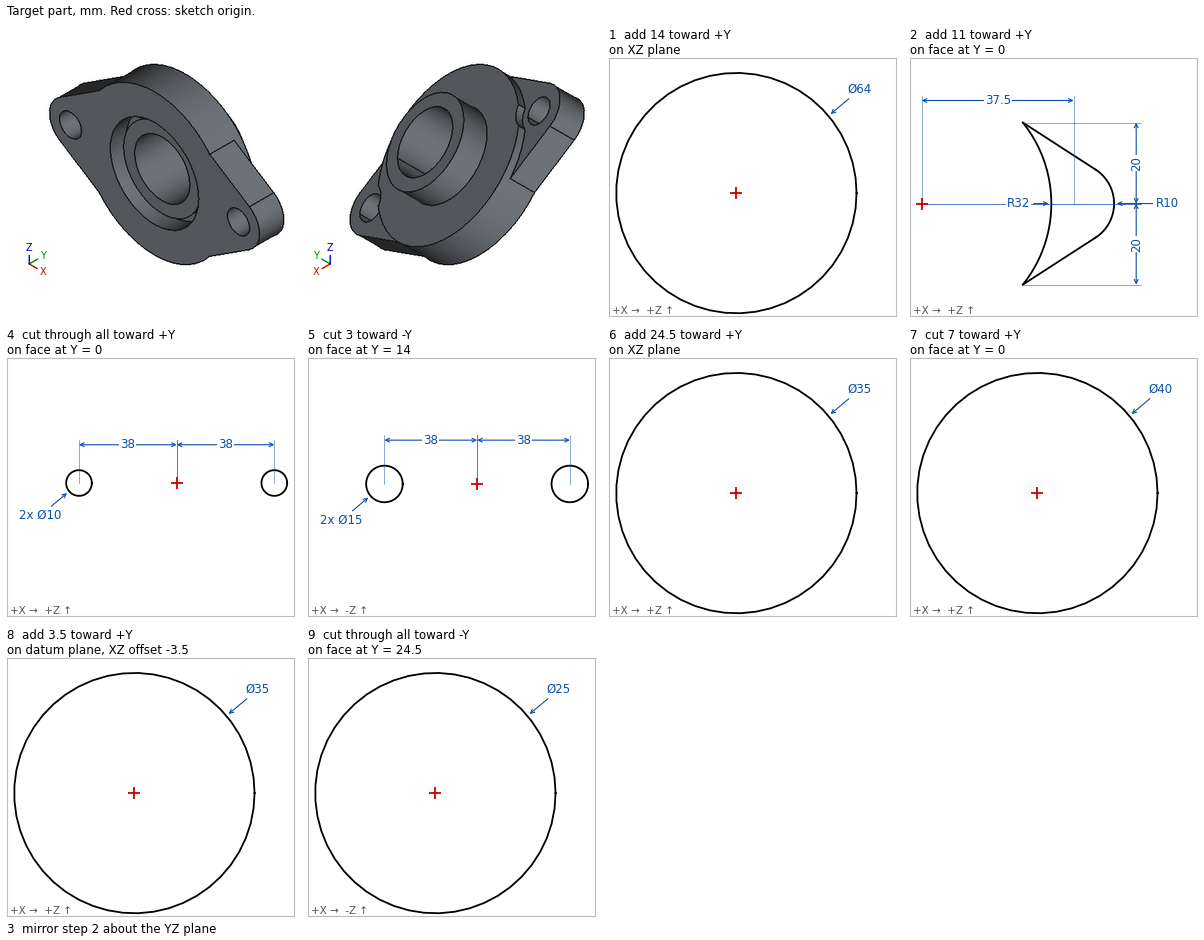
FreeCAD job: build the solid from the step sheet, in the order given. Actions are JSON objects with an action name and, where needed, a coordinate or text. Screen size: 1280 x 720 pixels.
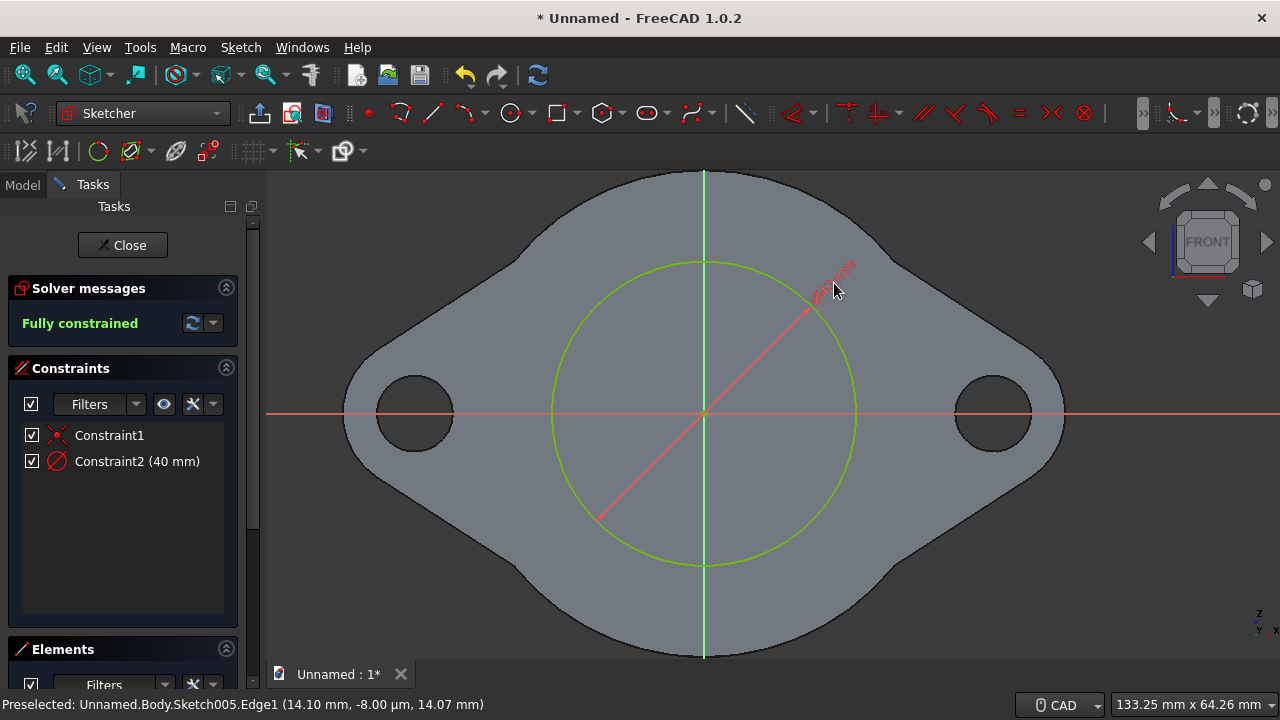
{"action": "left_click", "coordinate": [123, 245]}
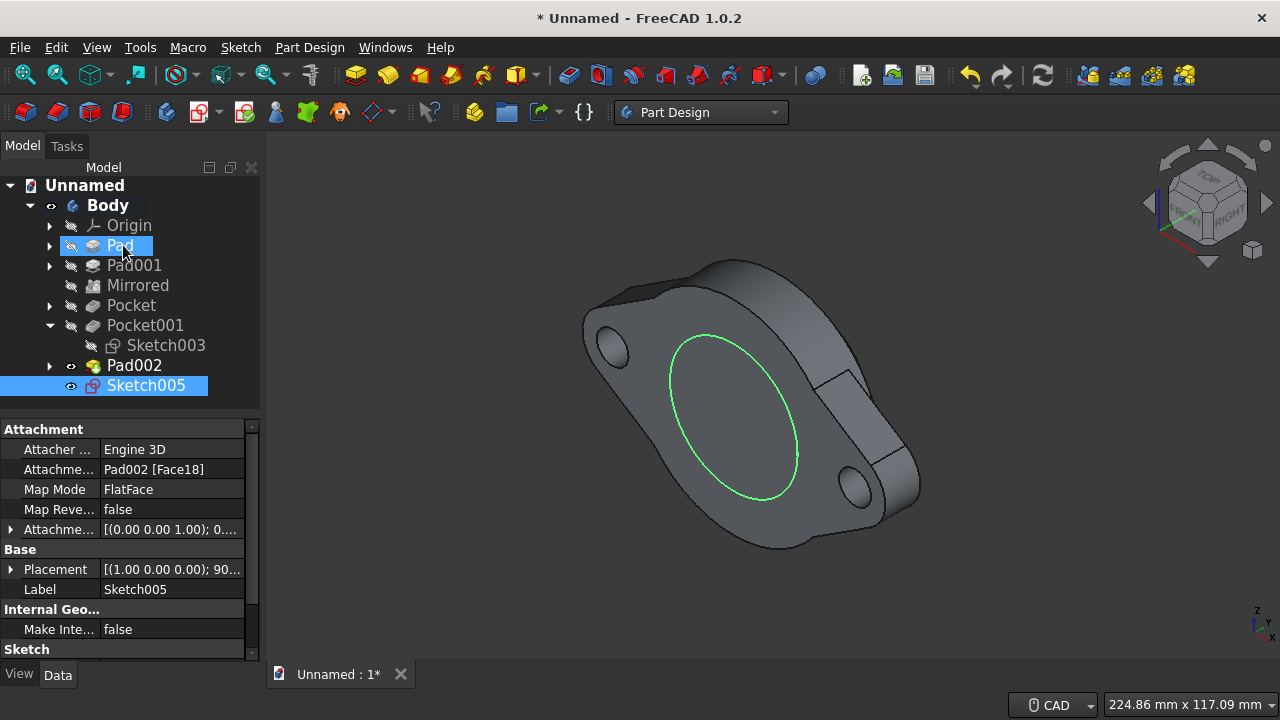
{"action": "left_click", "coordinate": [570, 76]}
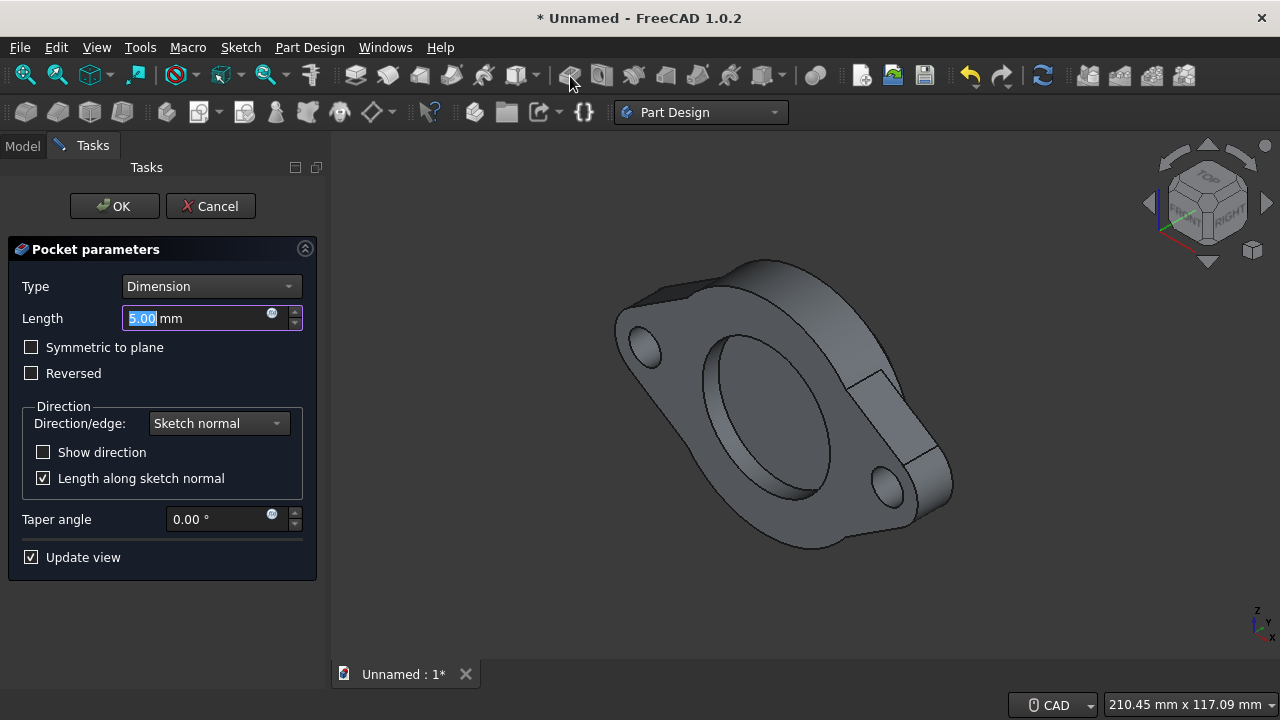
{"action": "type", "text": "7"}
{"action": "key", "text": "Tab"}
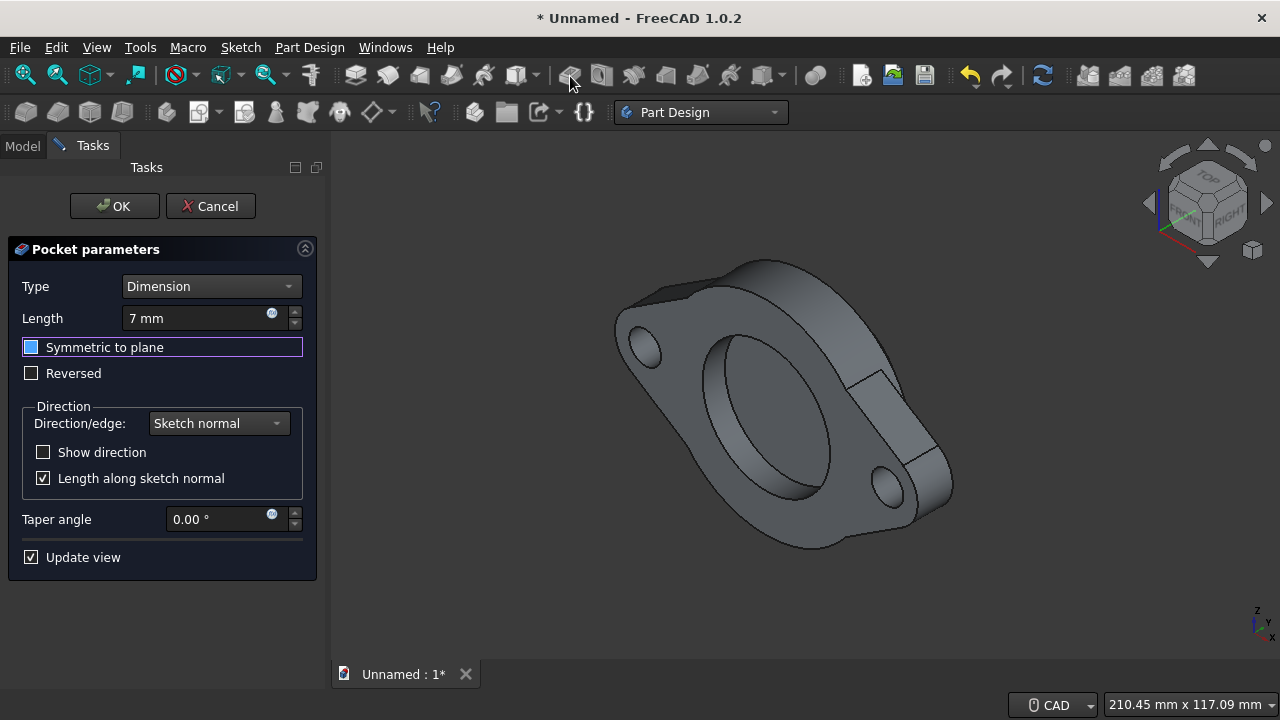
{"action": "left_click", "coordinate": [115, 206]}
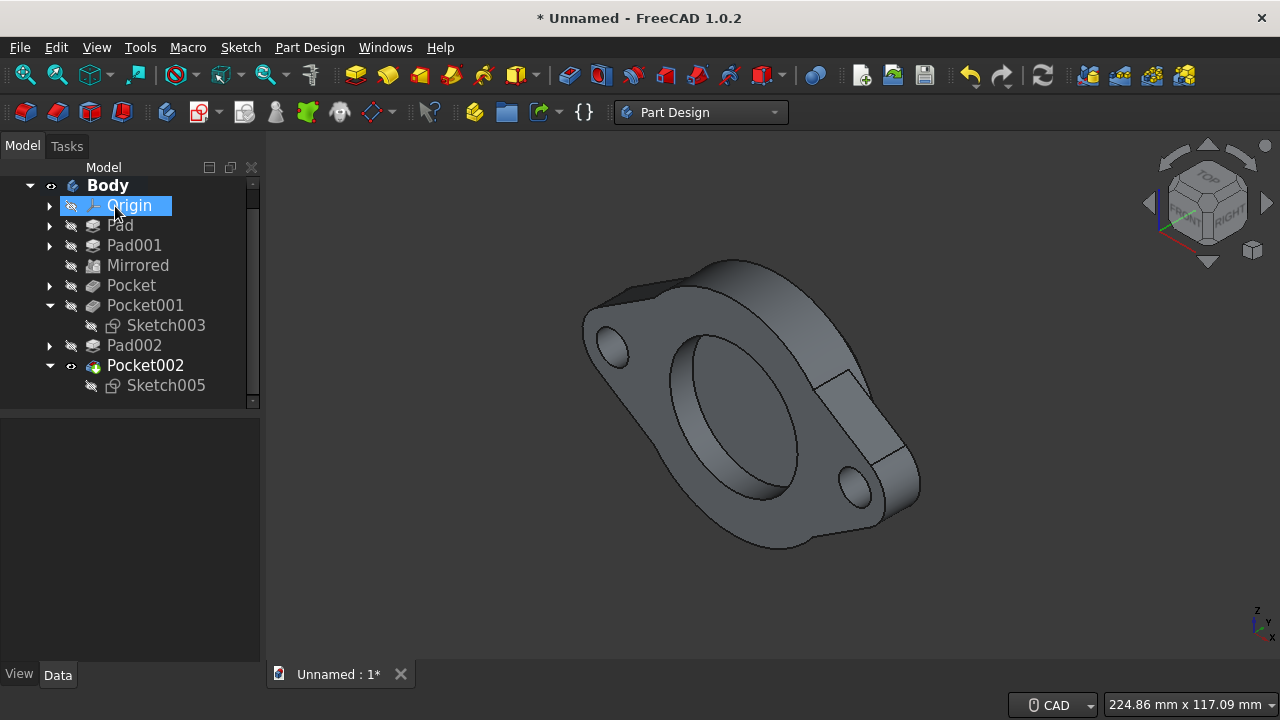
{"action": "left_click", "coordinate": [50, 206]}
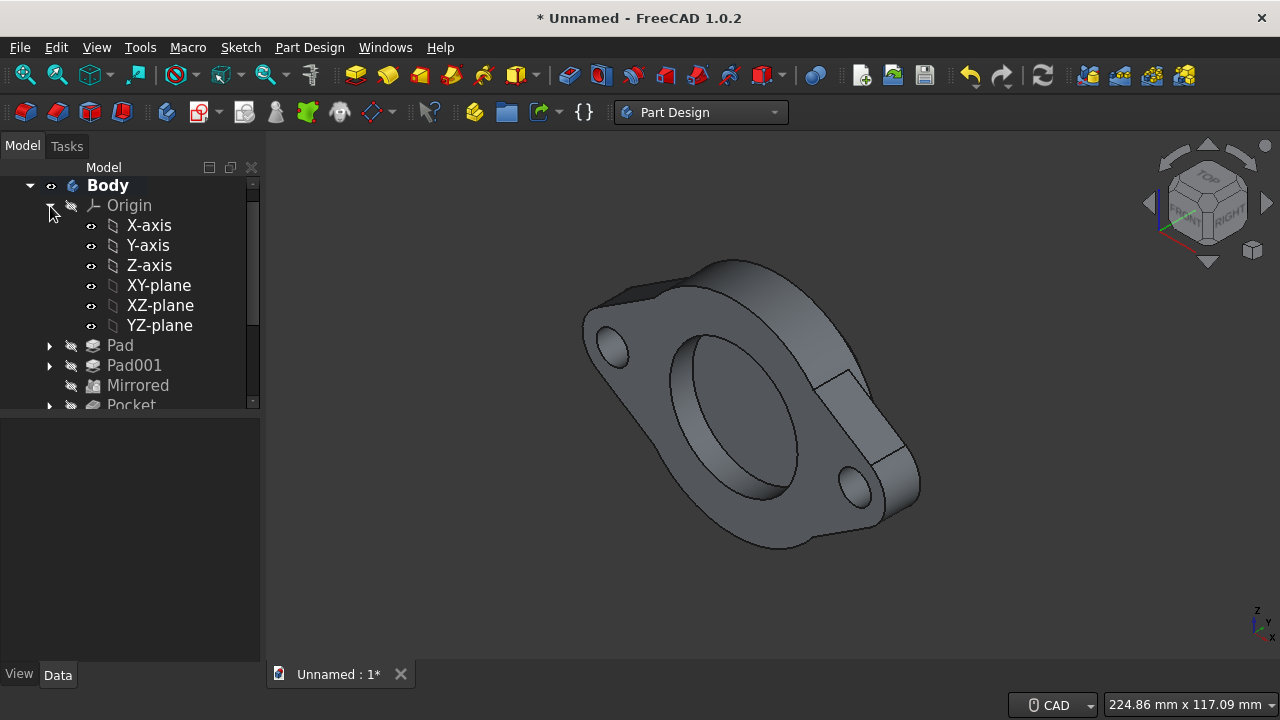
{"action": "left_click", "coordinate": [136, 306]}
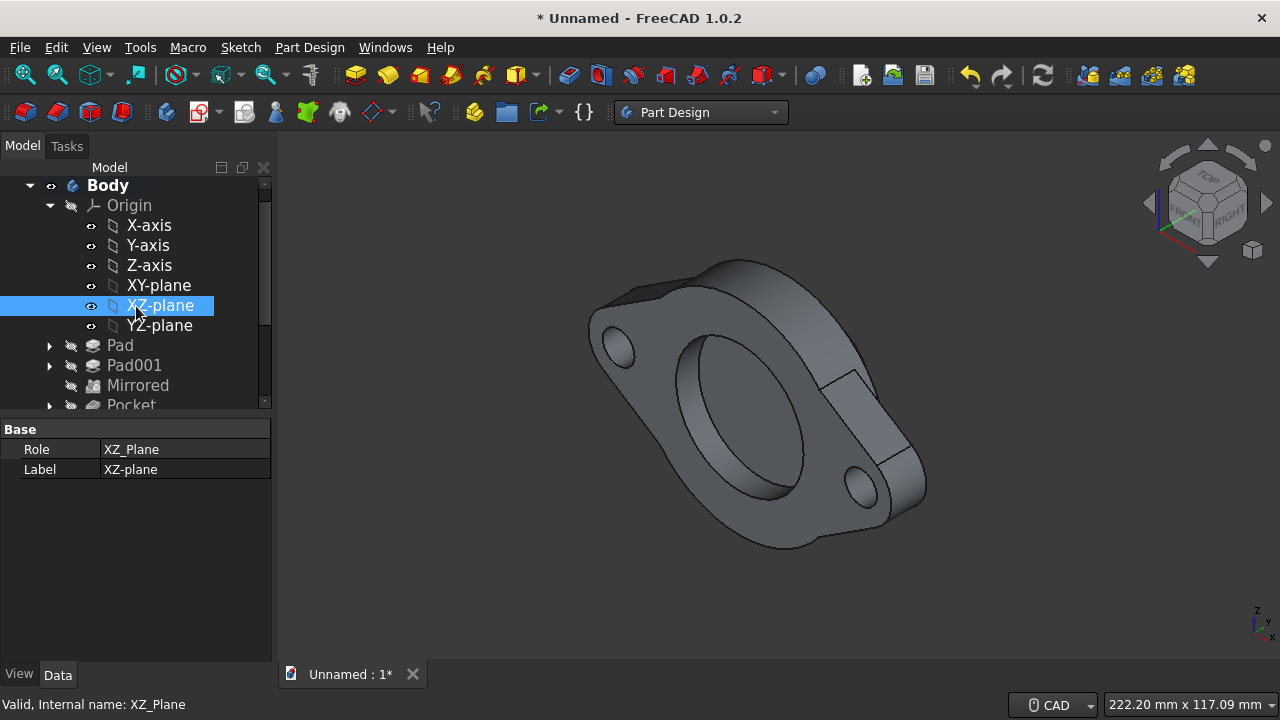
{"action": "left_click", "coordinate": [372, 112]}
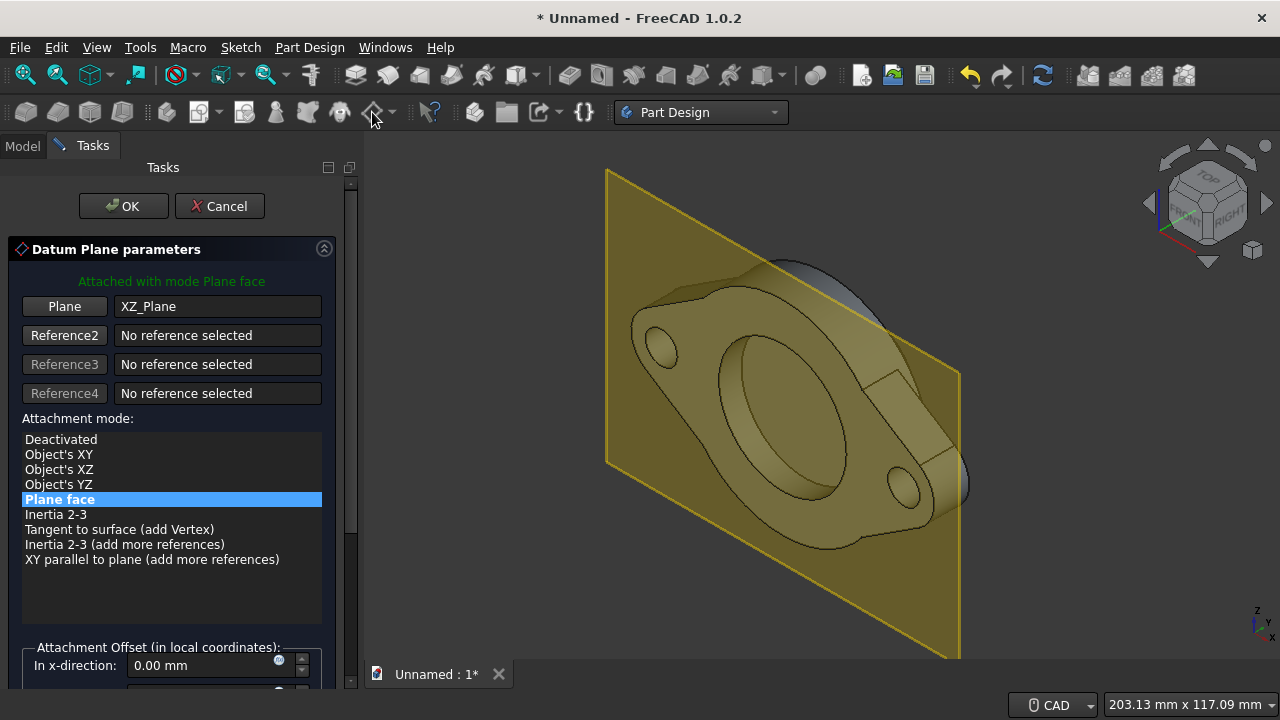
{"action": "scroll", "coordinate": [351, 432], "scroll_direction": "down", "scroll_amount": 2}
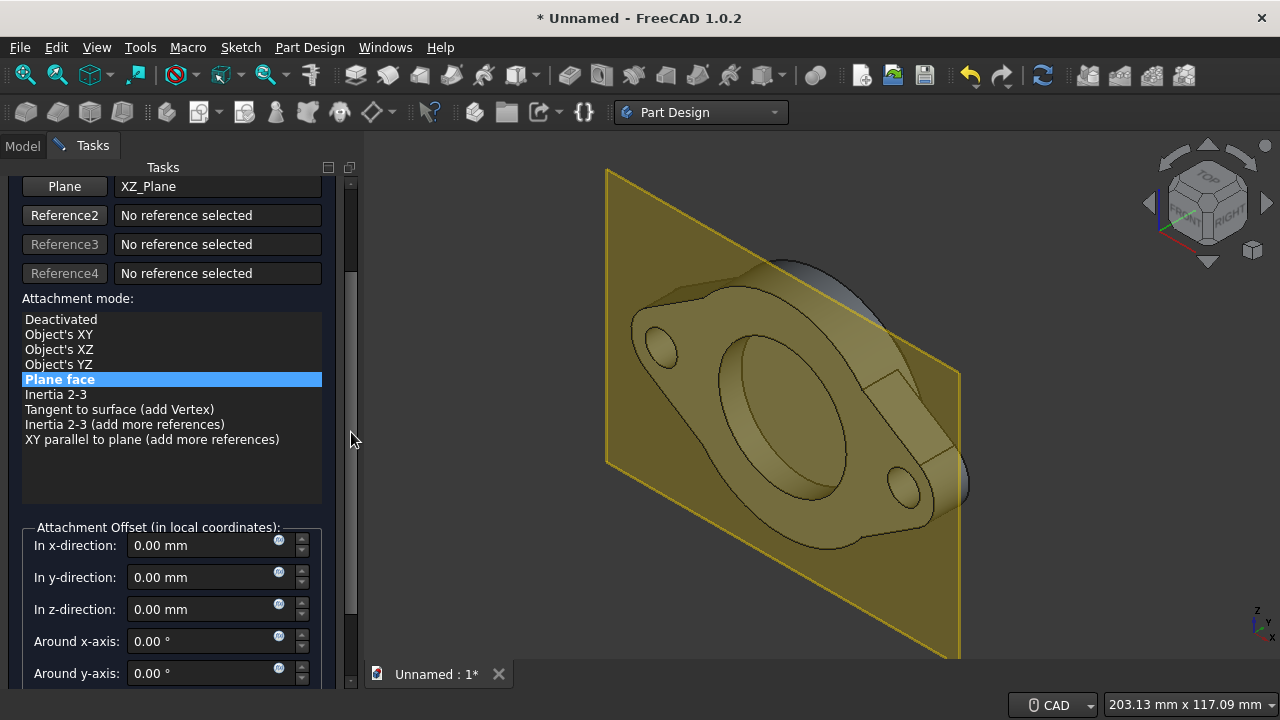
{"action": "triple_click", "coordinate": [210, 609]}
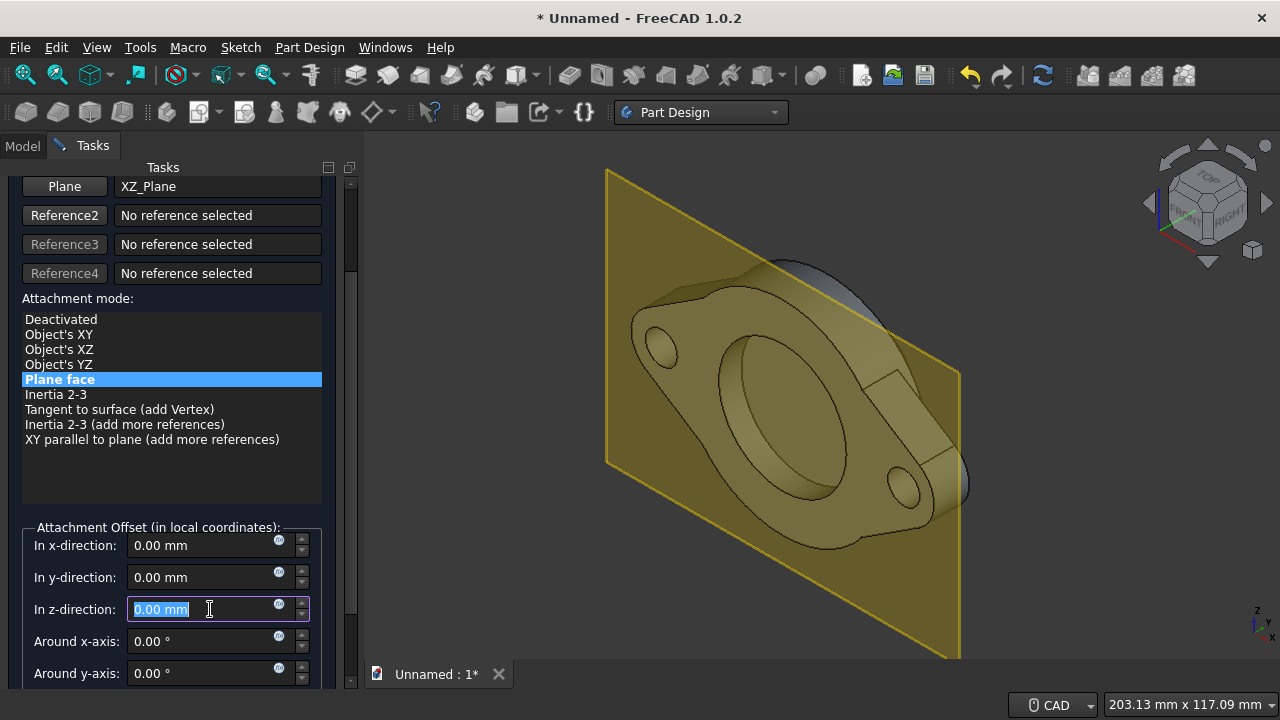
{"action": "type", "text": "-3.5"}
{"action": "key", "text": "Tab"}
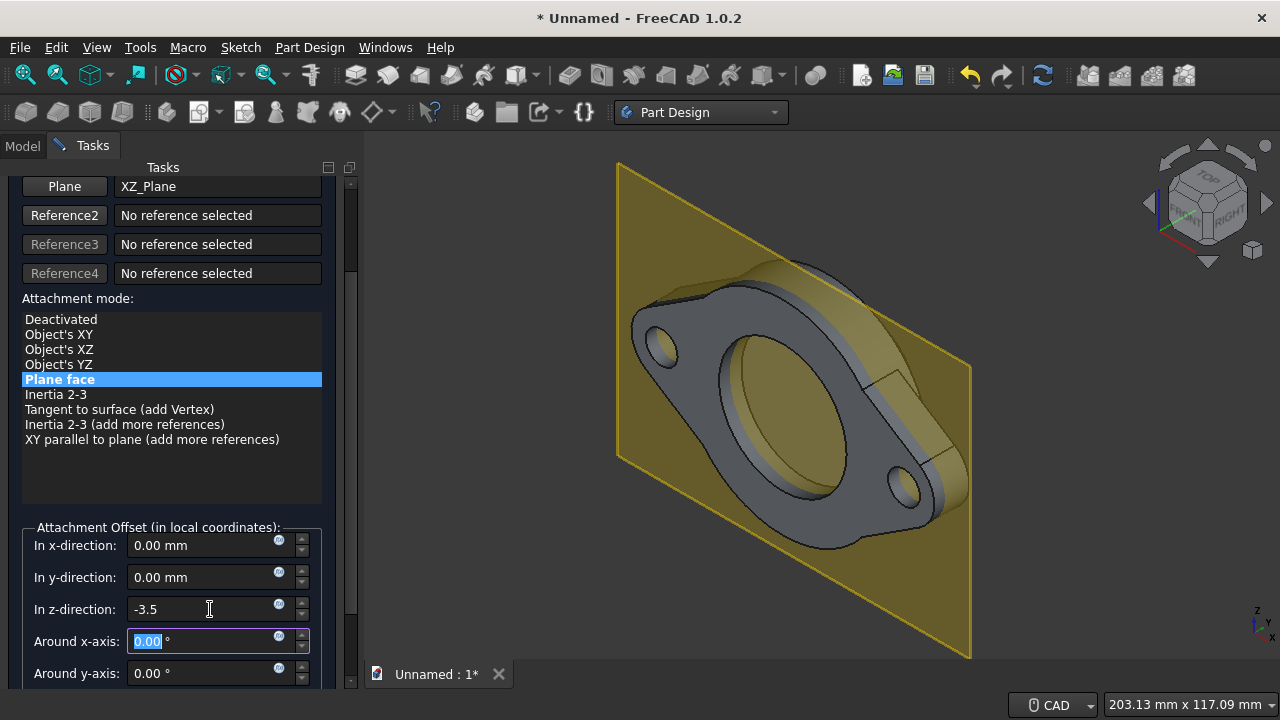
{"action": "scroll", "coordinate": [351, 432], "scroll_direction": "up", "scroll_amount": 3}